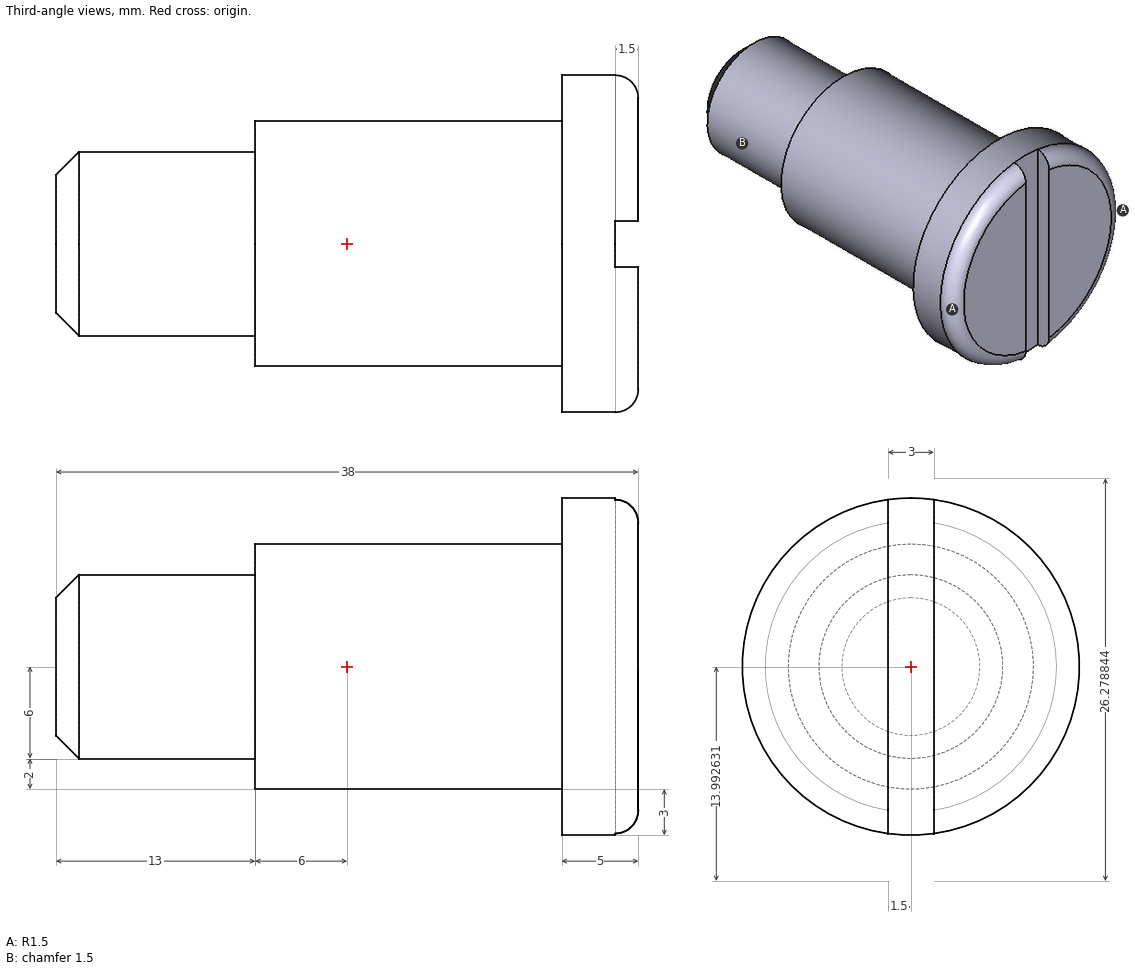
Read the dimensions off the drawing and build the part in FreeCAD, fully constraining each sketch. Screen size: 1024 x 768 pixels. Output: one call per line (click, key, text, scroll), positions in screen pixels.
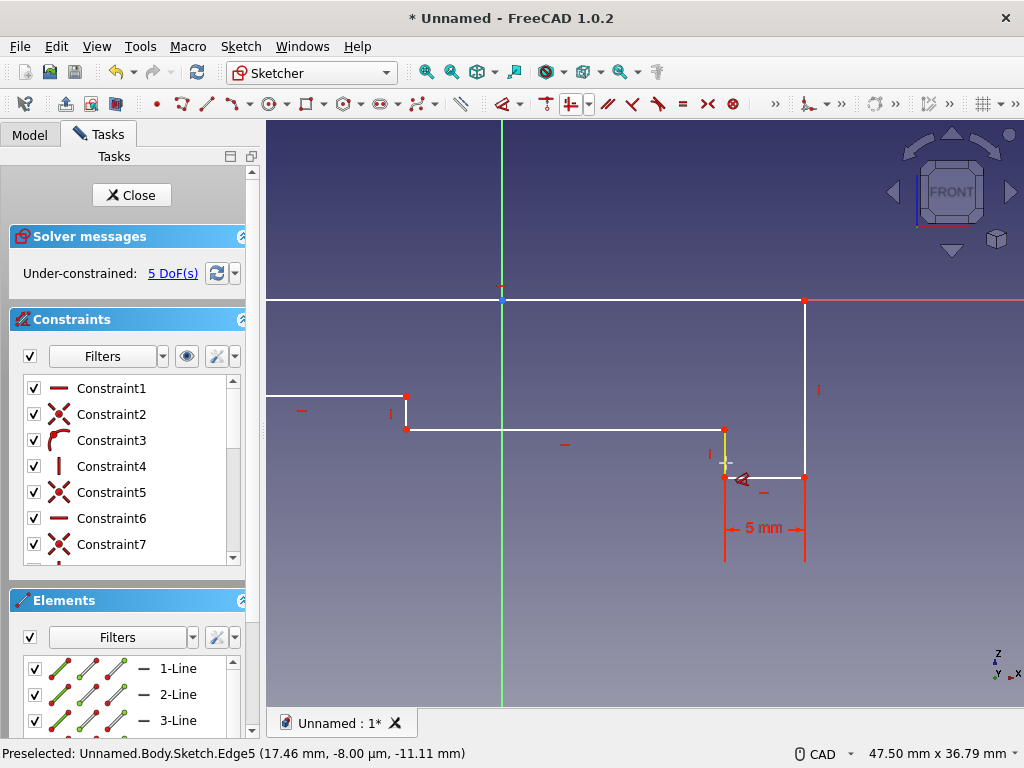
click(725, 463)
click(759, 454)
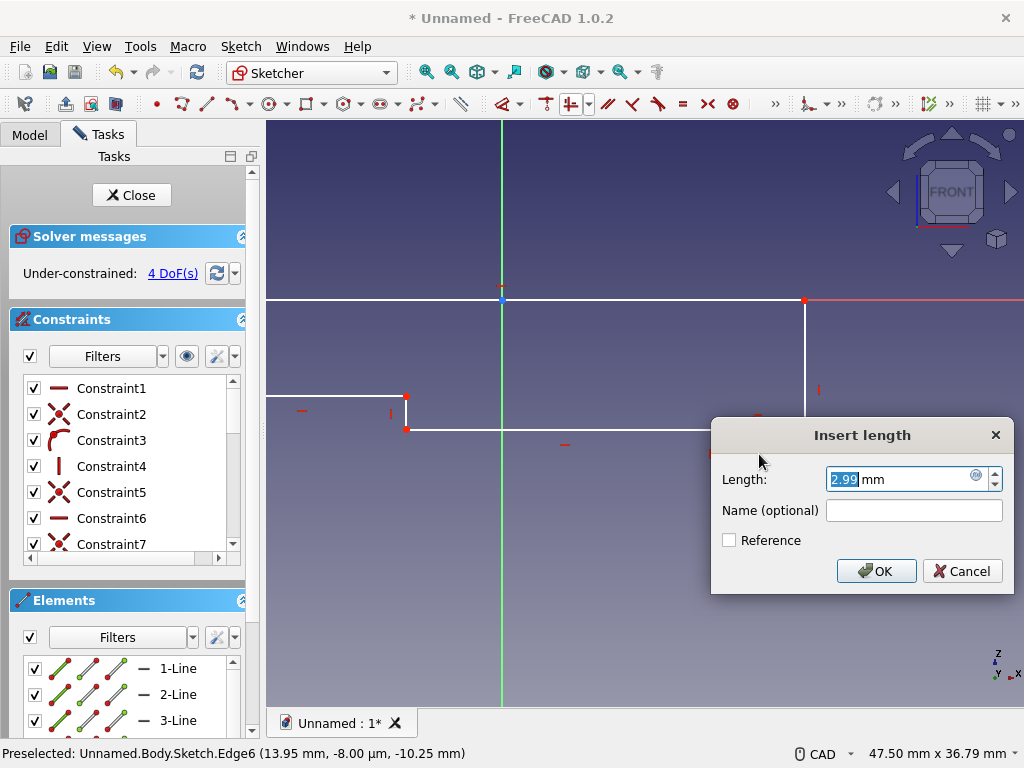
text(3)
key(Return)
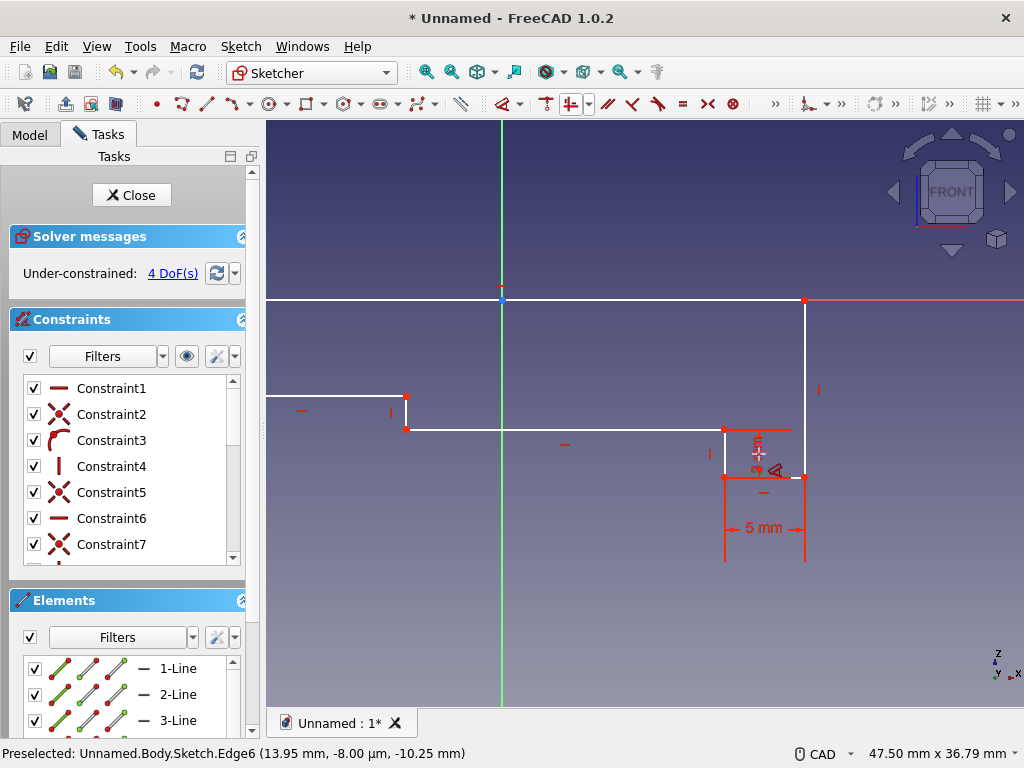
scroll(406, 420, up, 2)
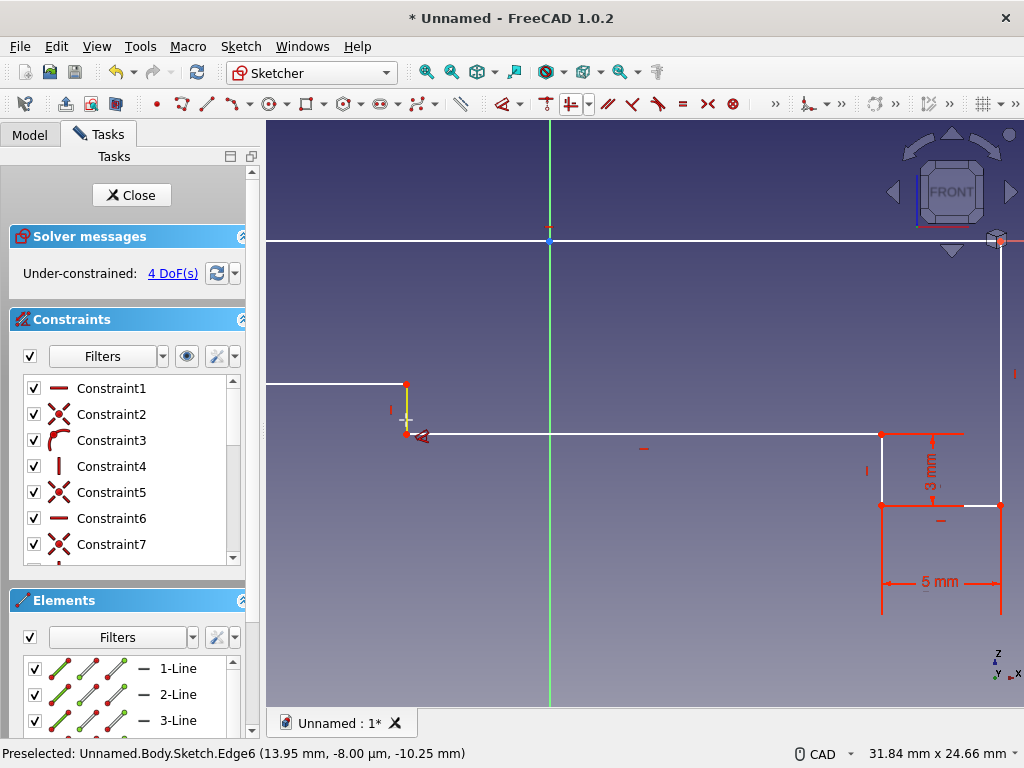
click(407, 419)
click(373, 409)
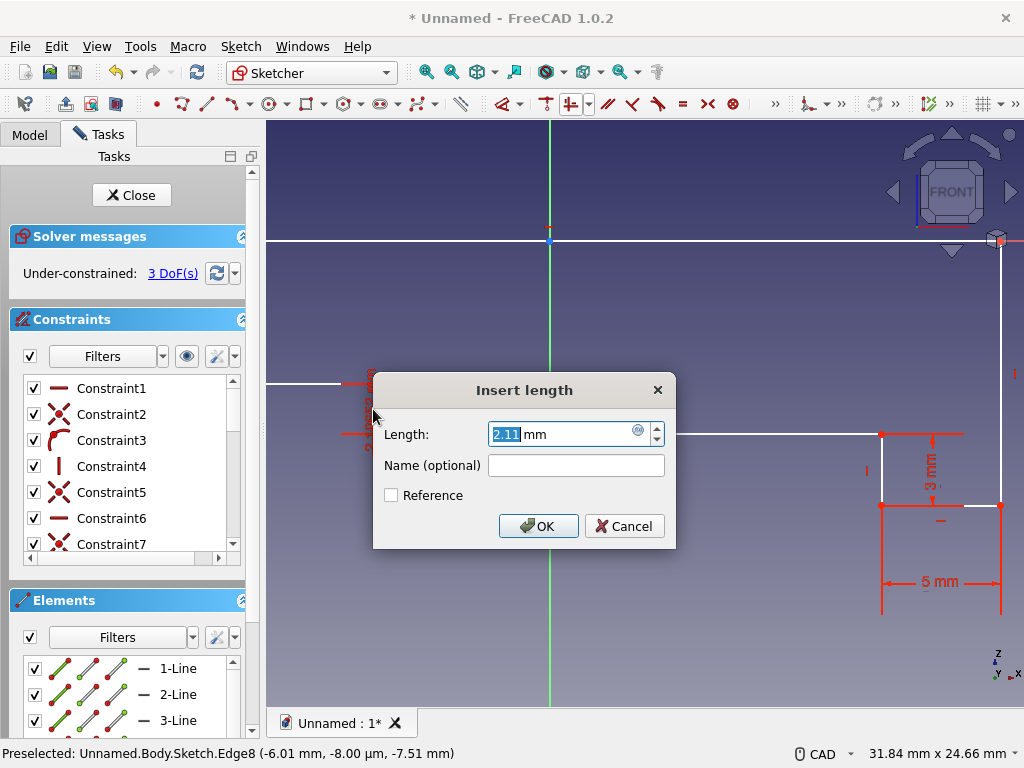
text(2)
key(Return)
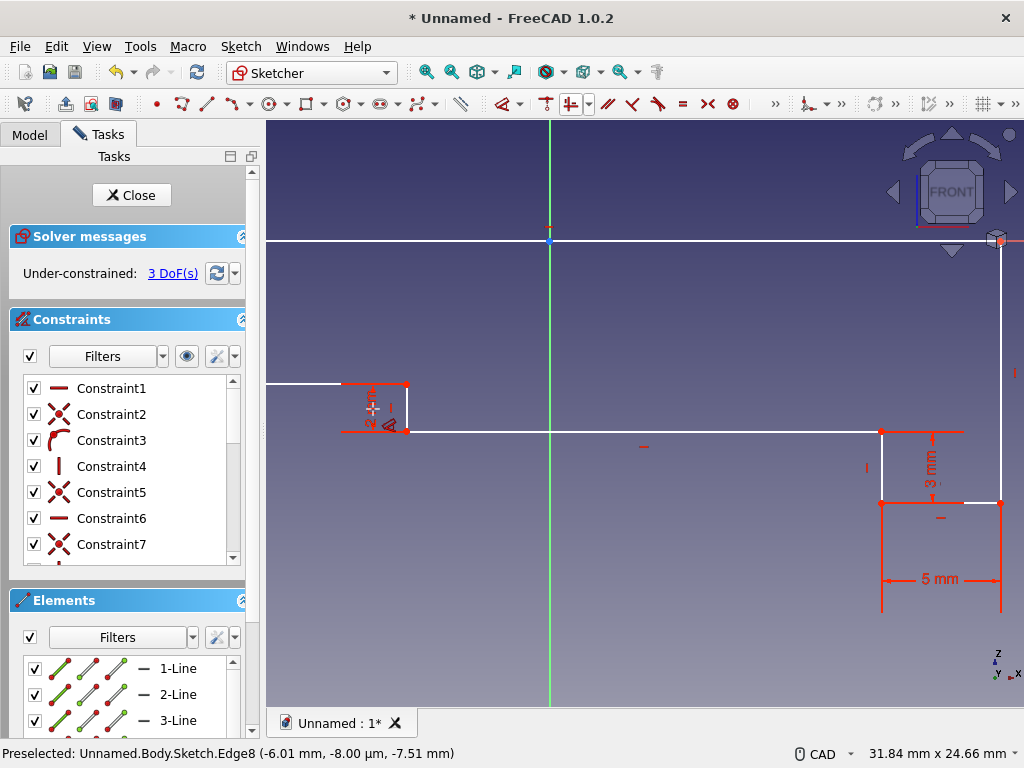
click(314, 384)
click(350, 350)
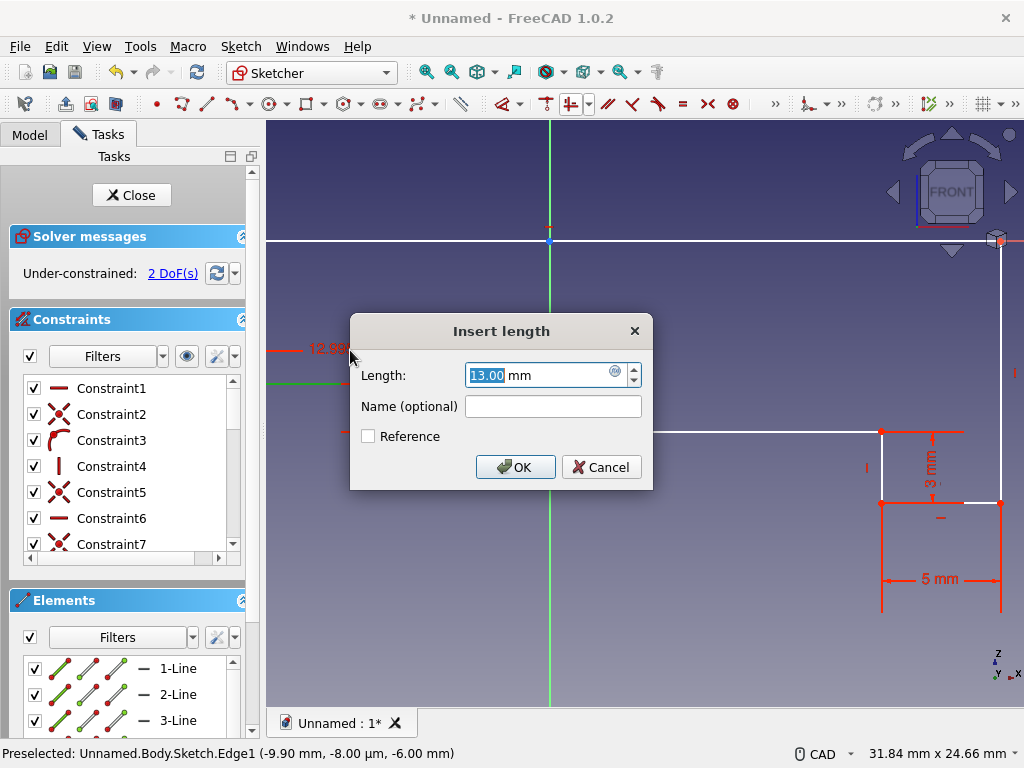
text(13)
key(Return)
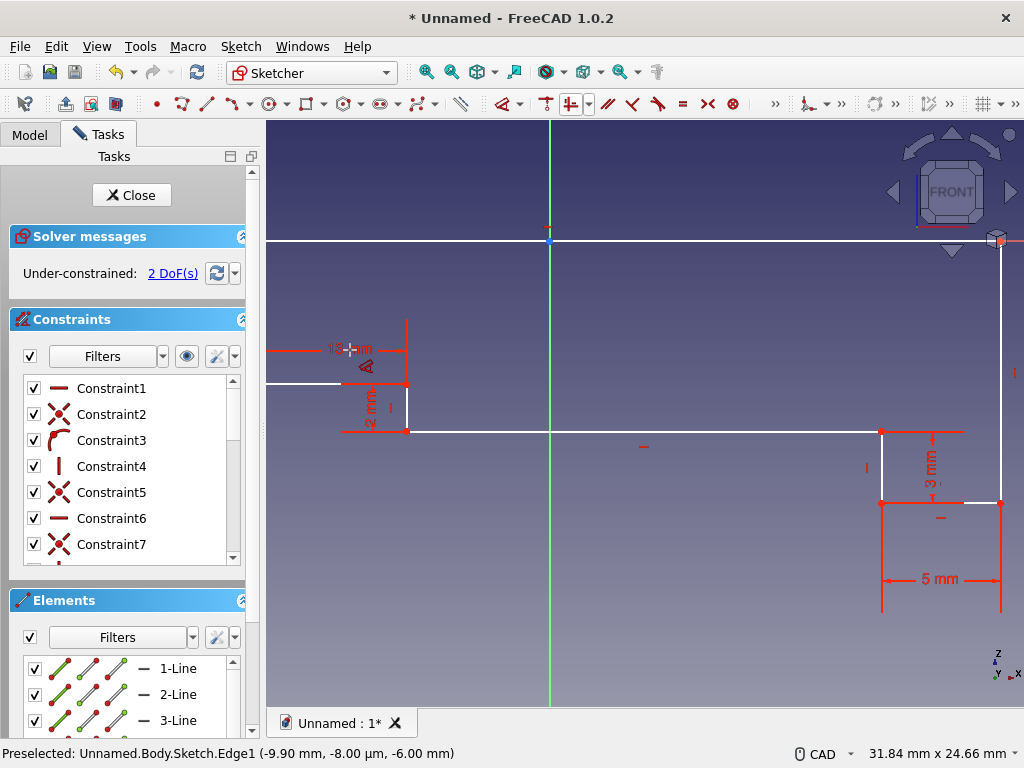
click(368, 241)
click(576, 207)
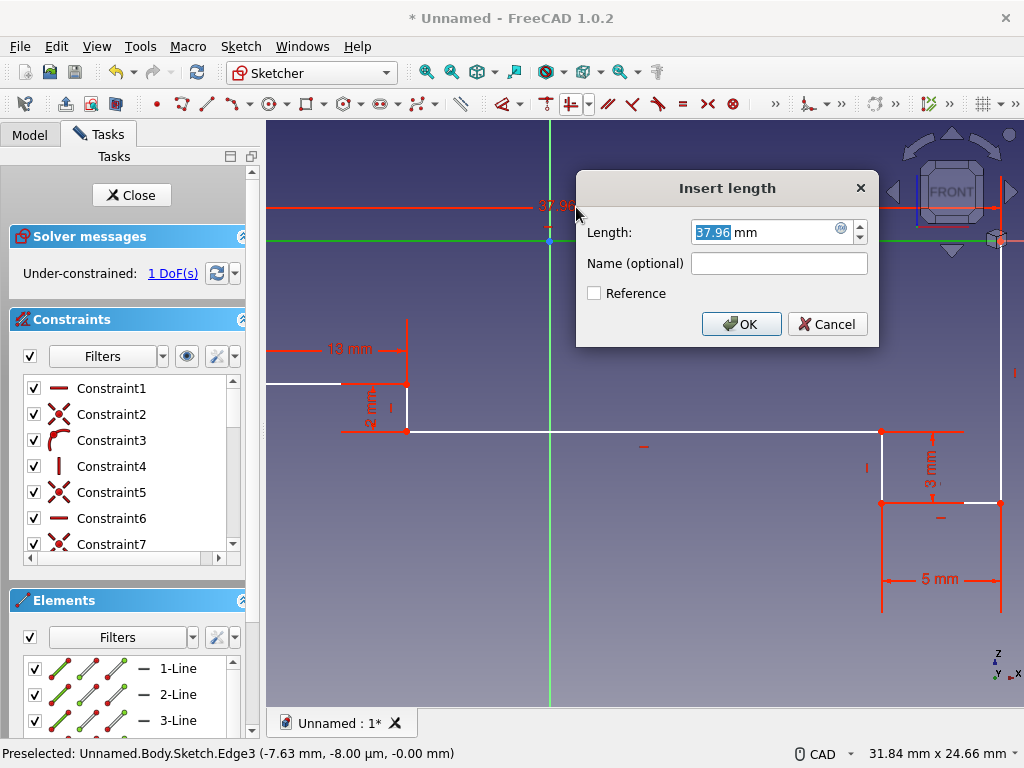
text(38)
key(Return)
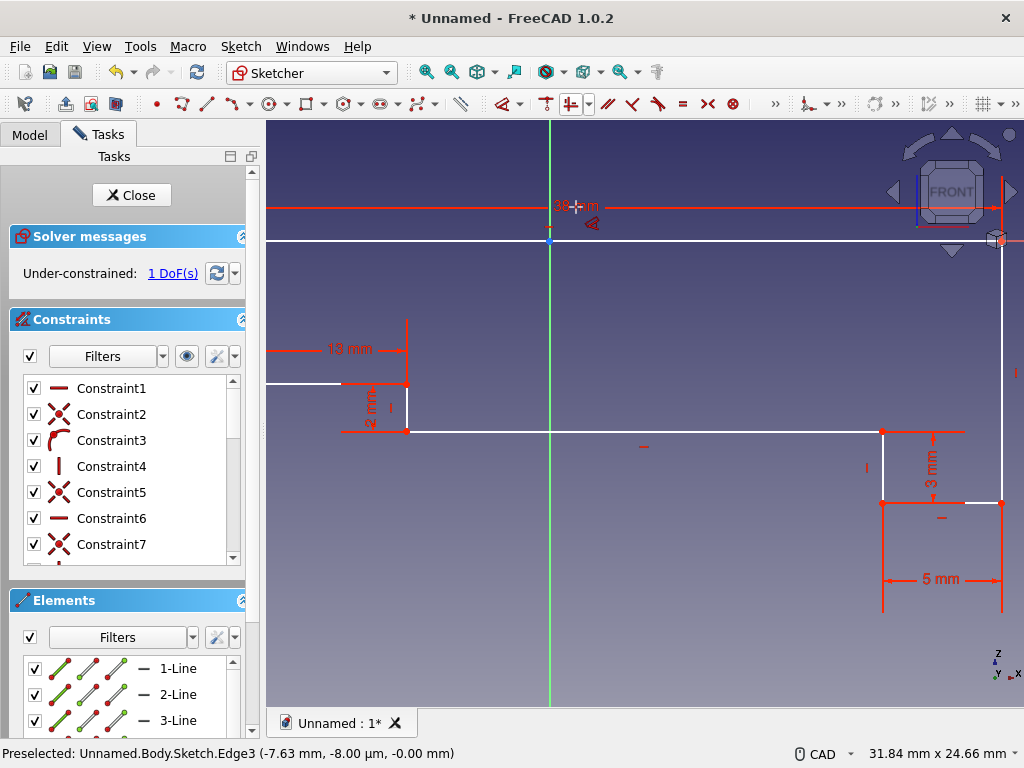
click(407, 384)
click(478, 207)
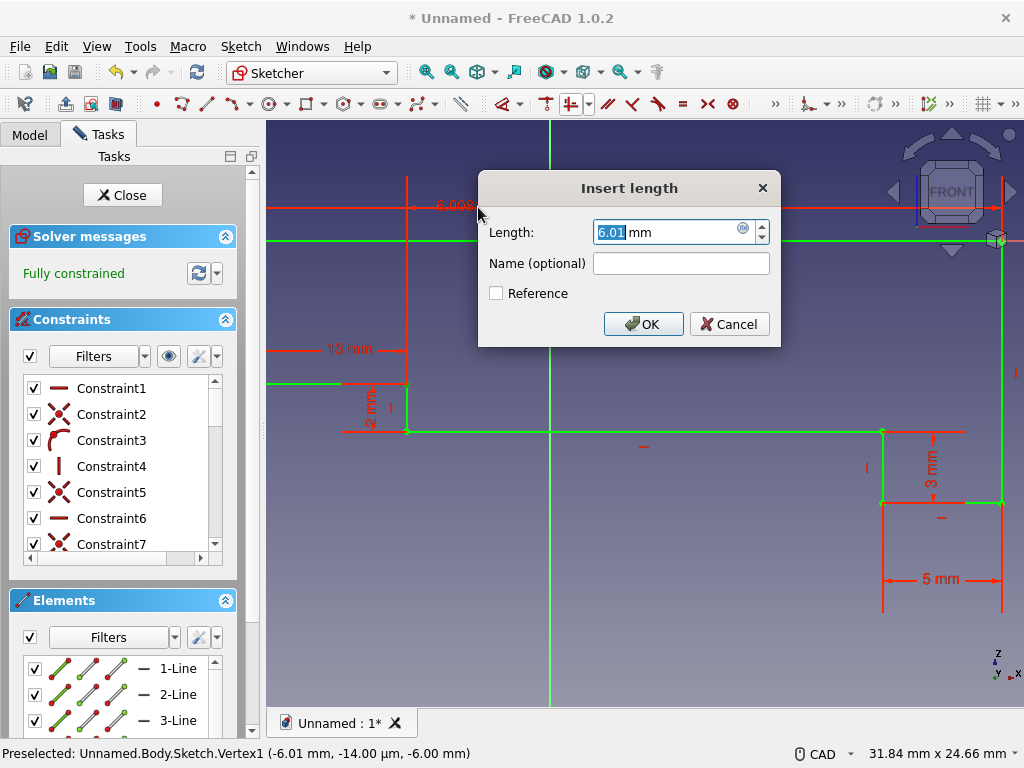
text(6)
key(Return)
key(Escape)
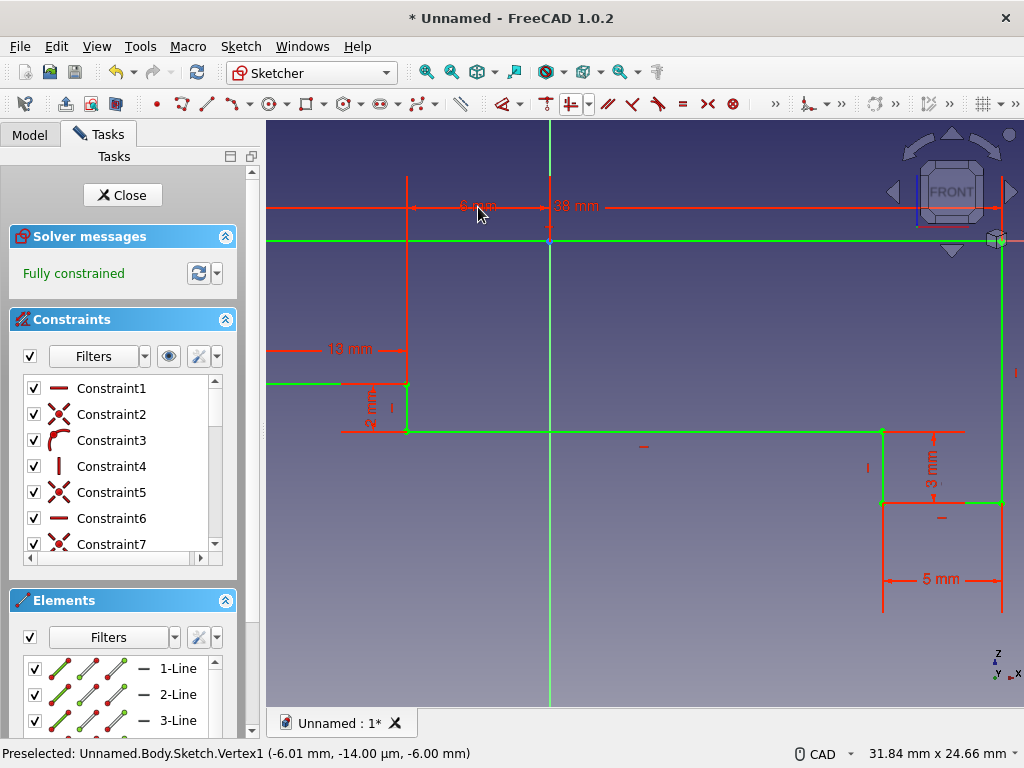
click(123, 195)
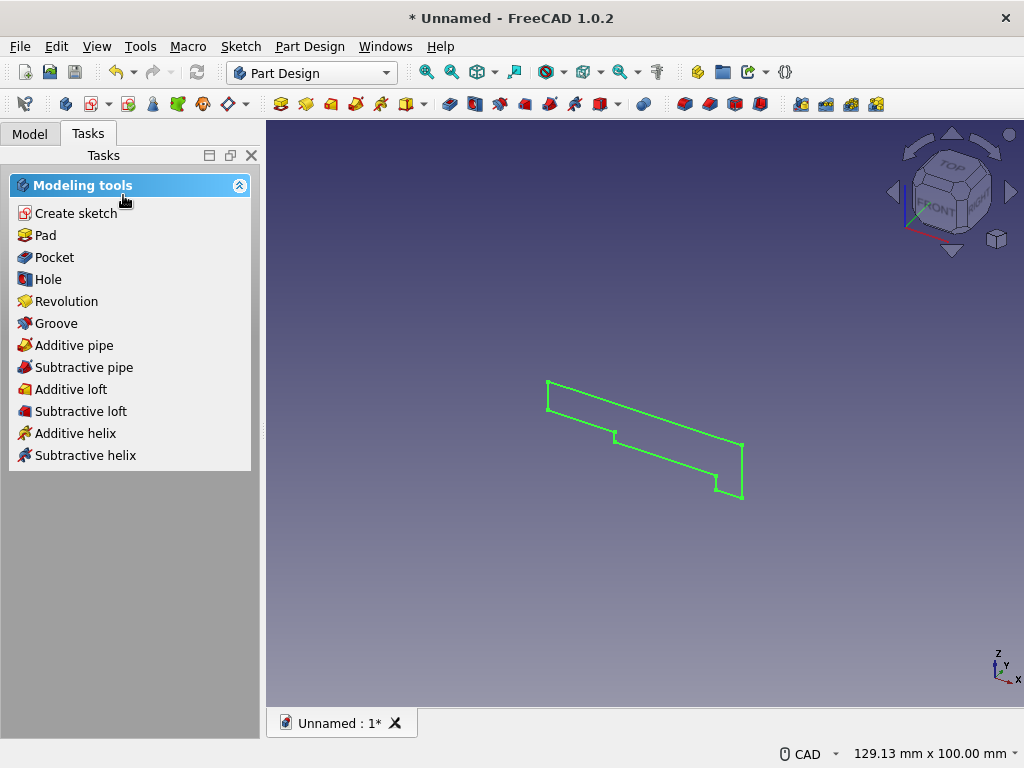
click(306, 104)